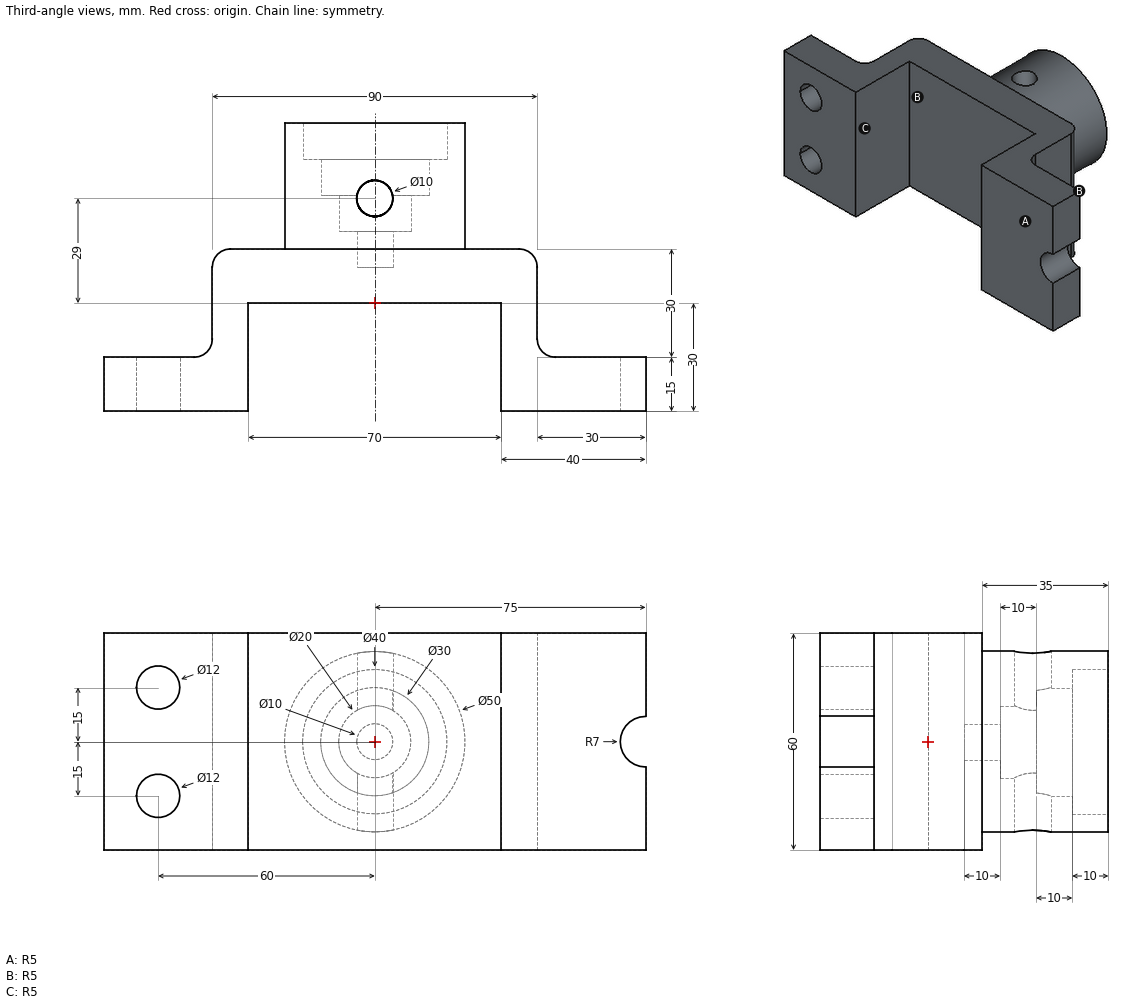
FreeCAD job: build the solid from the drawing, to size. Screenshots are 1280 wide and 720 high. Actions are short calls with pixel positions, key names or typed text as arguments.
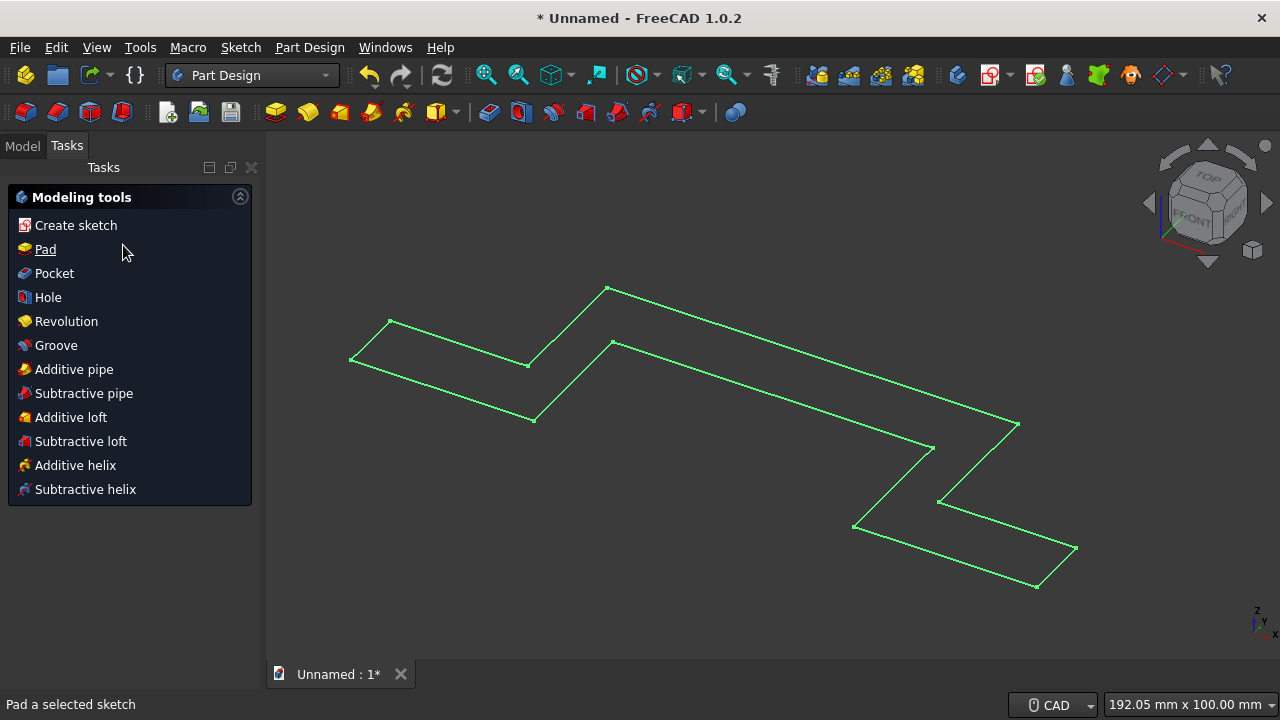
click(276, 112)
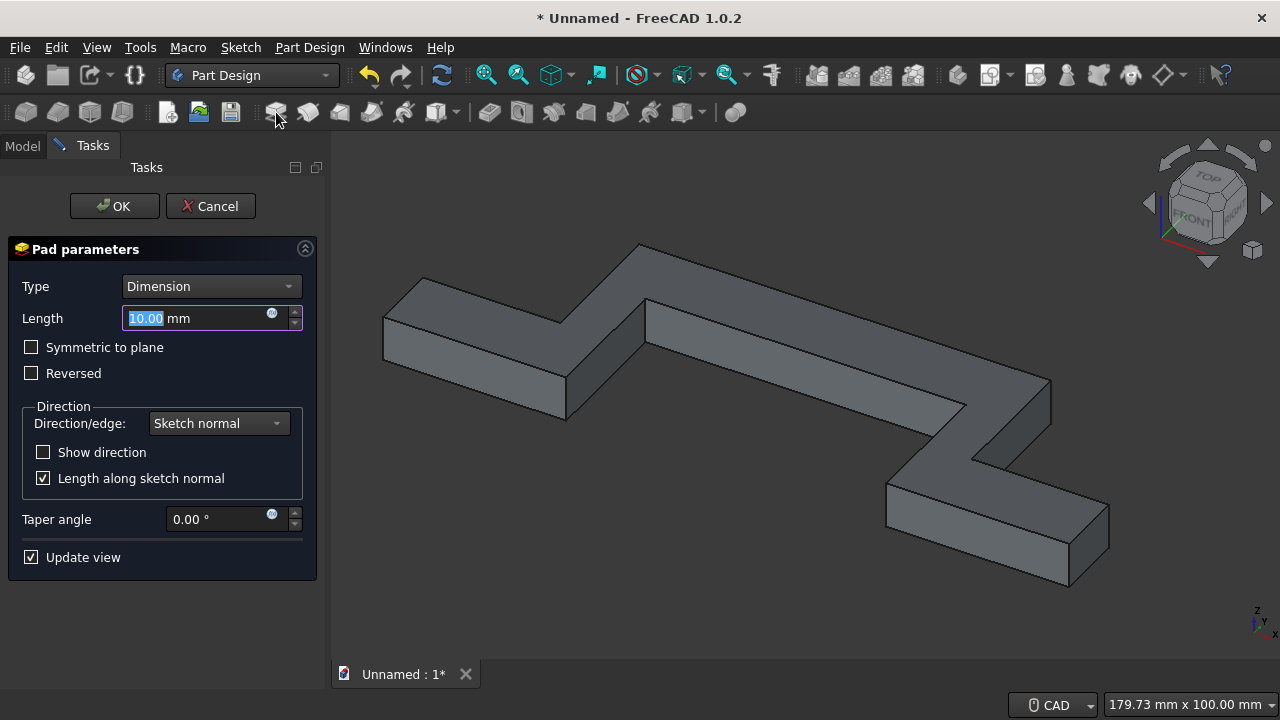
text(60)
key(Tab)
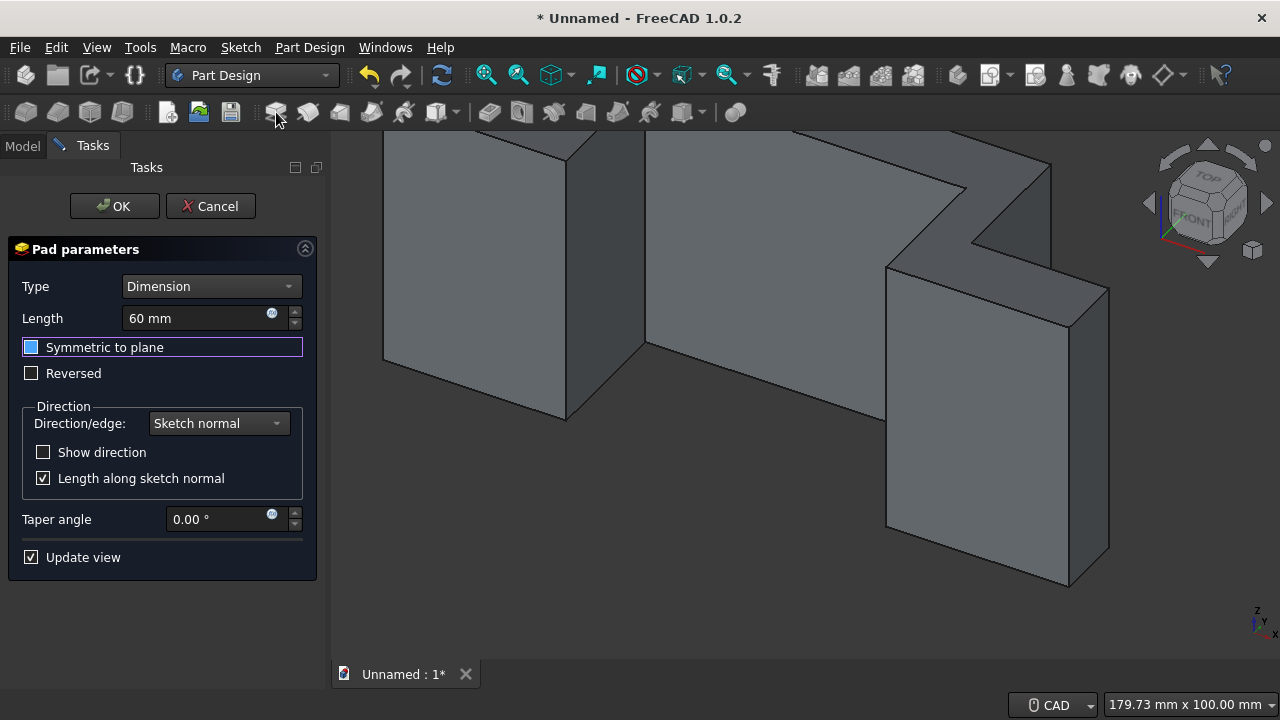
click(30, 347)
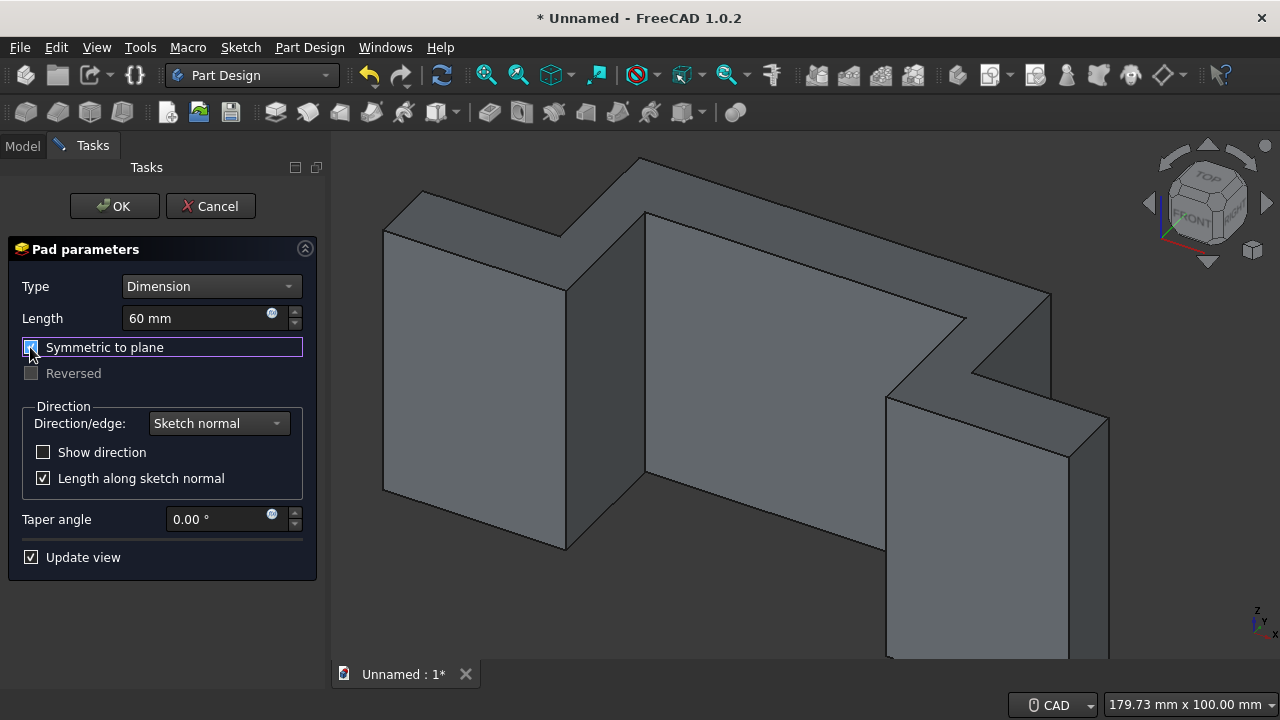
click(115, 206)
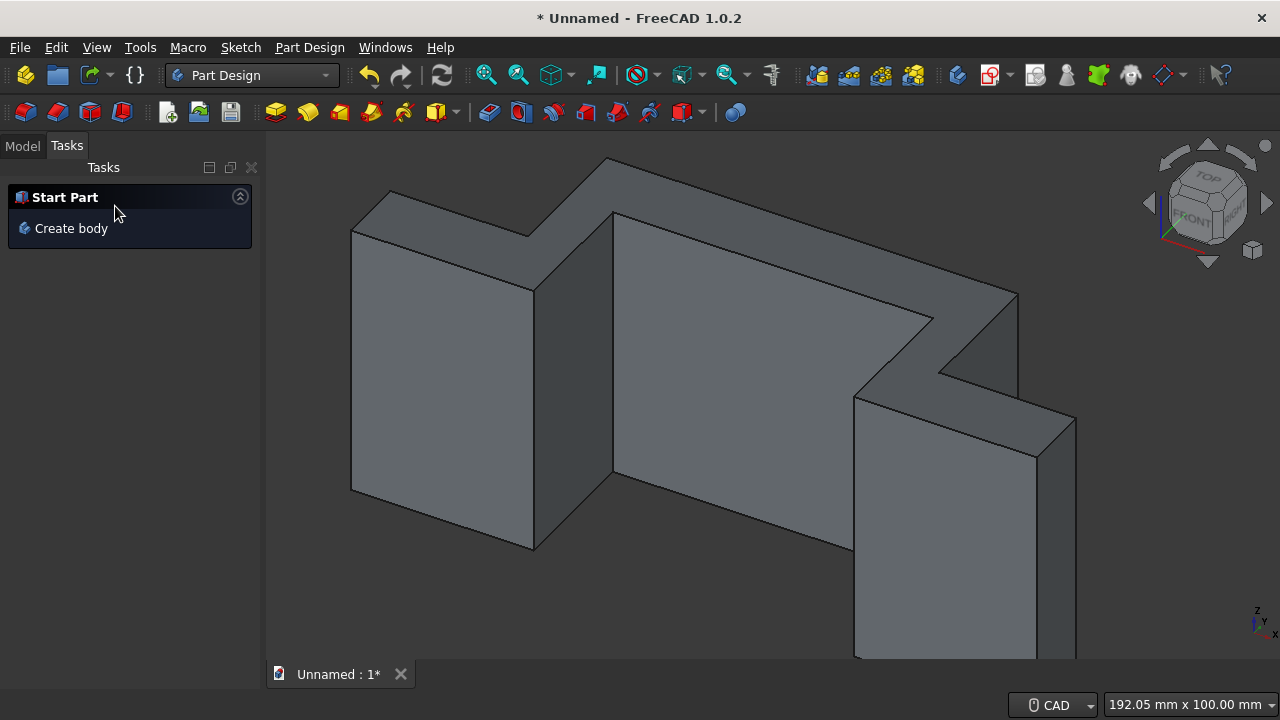
click(488, 76)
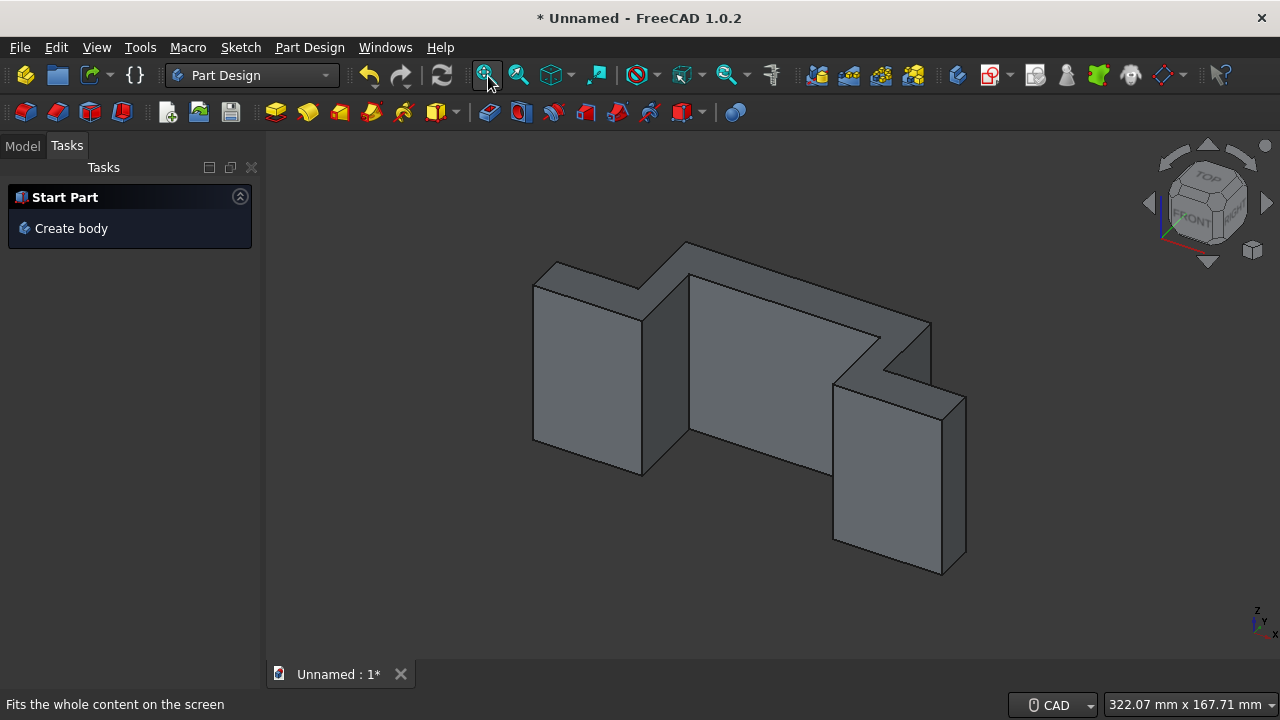
key(4)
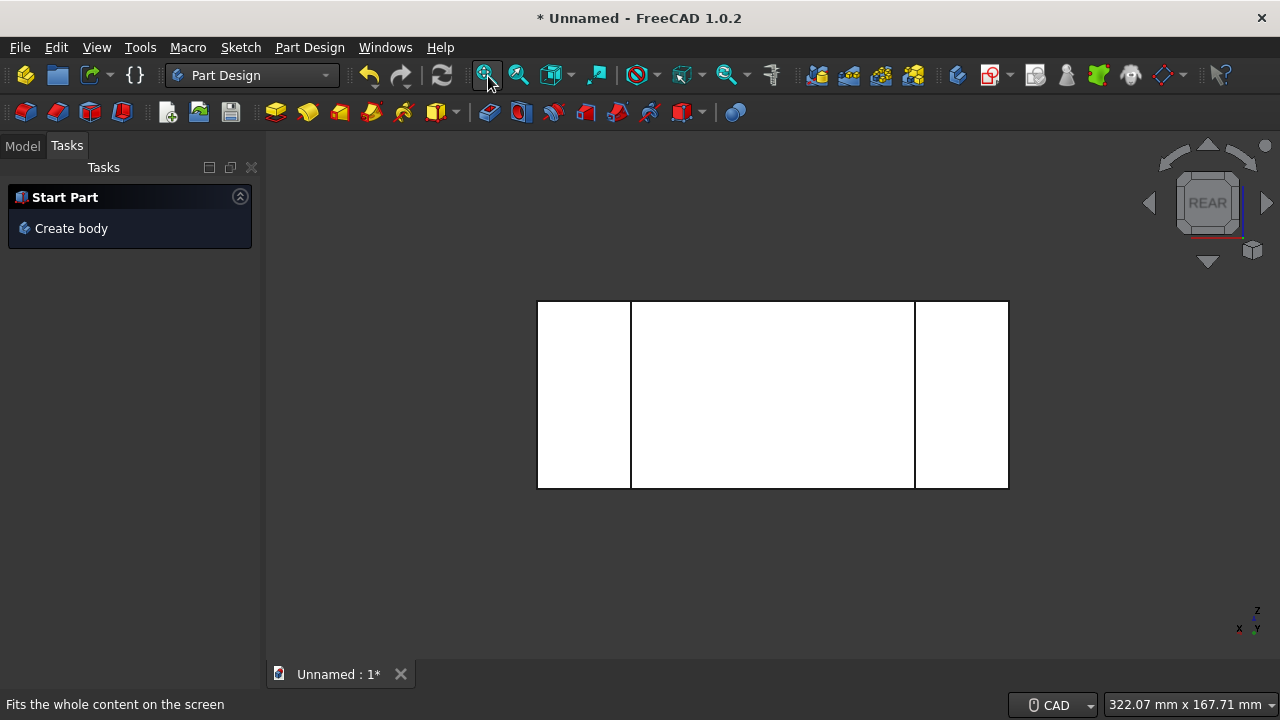
click(962, 367)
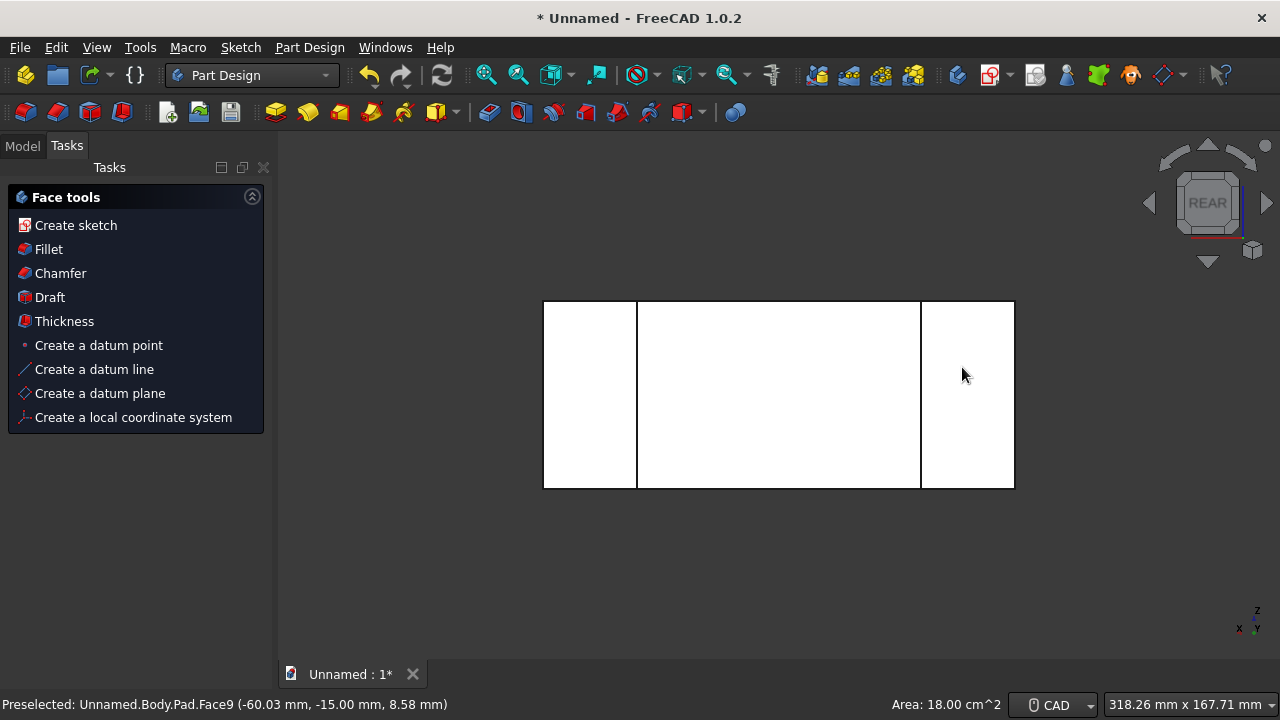
click(990, 76)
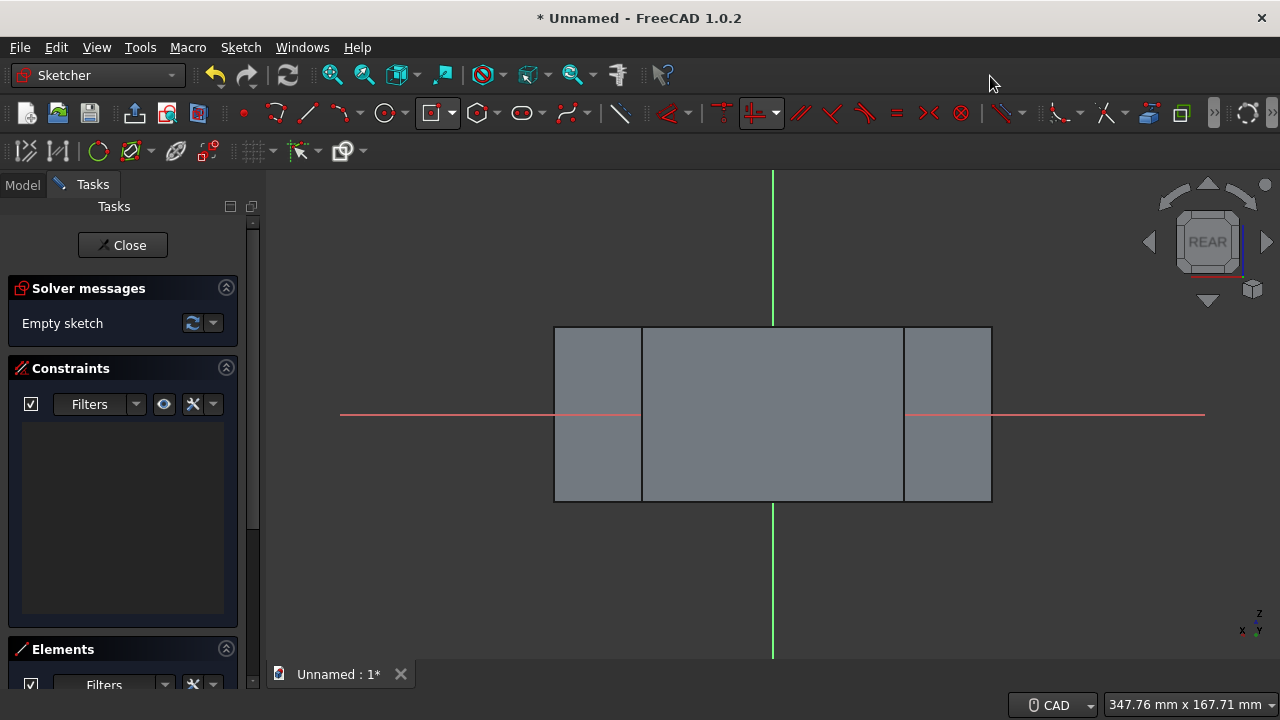
scroll(978, 464, up, 11)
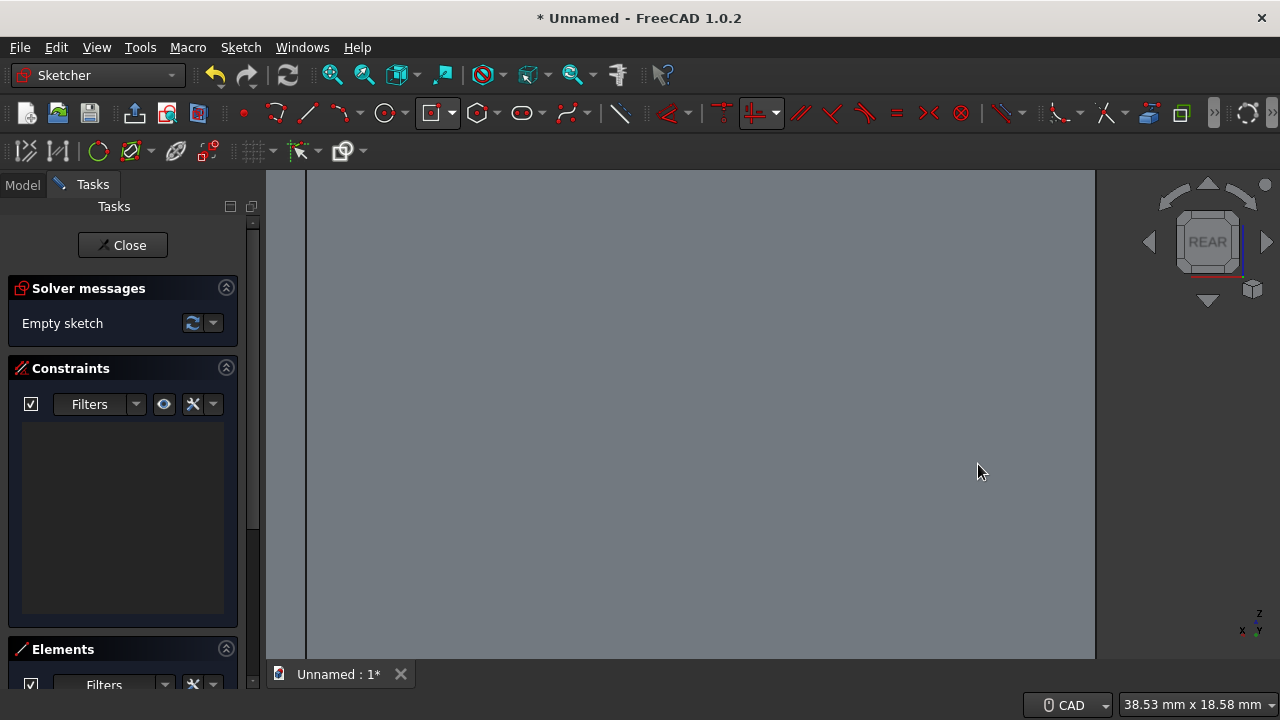
click(386, 114)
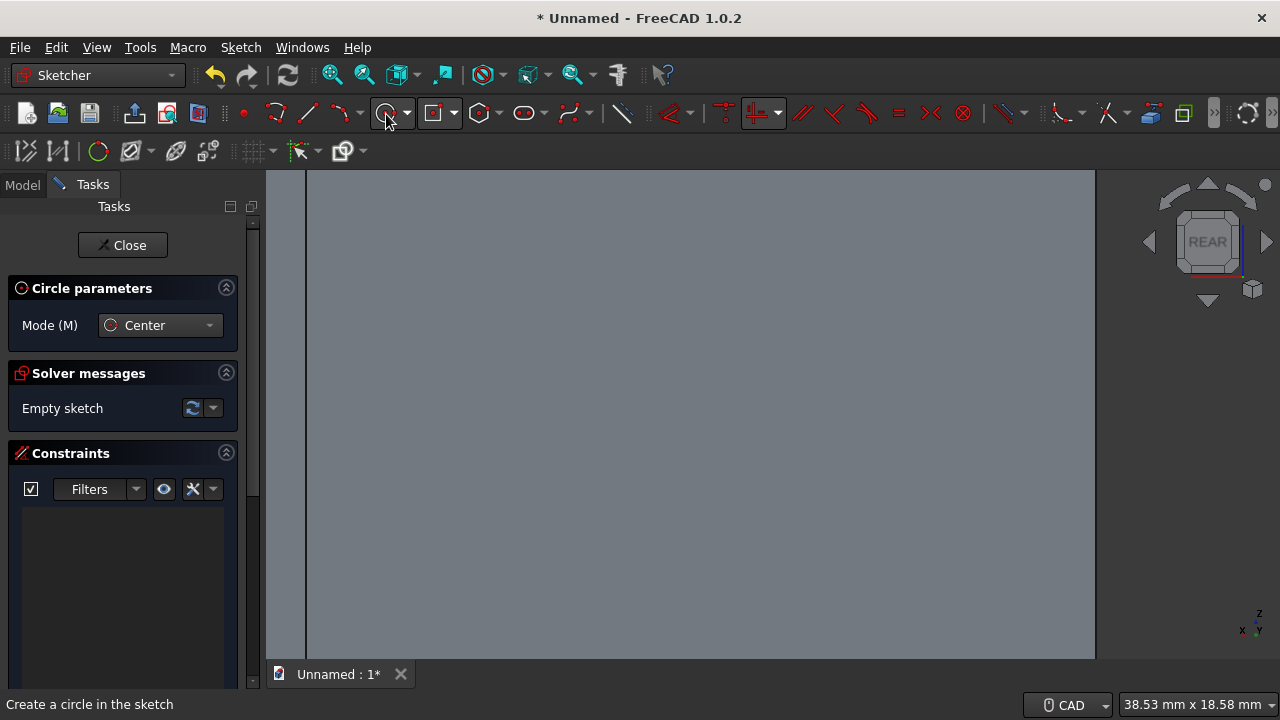
click(701, 407)
click(813, 296)
key(Escape)